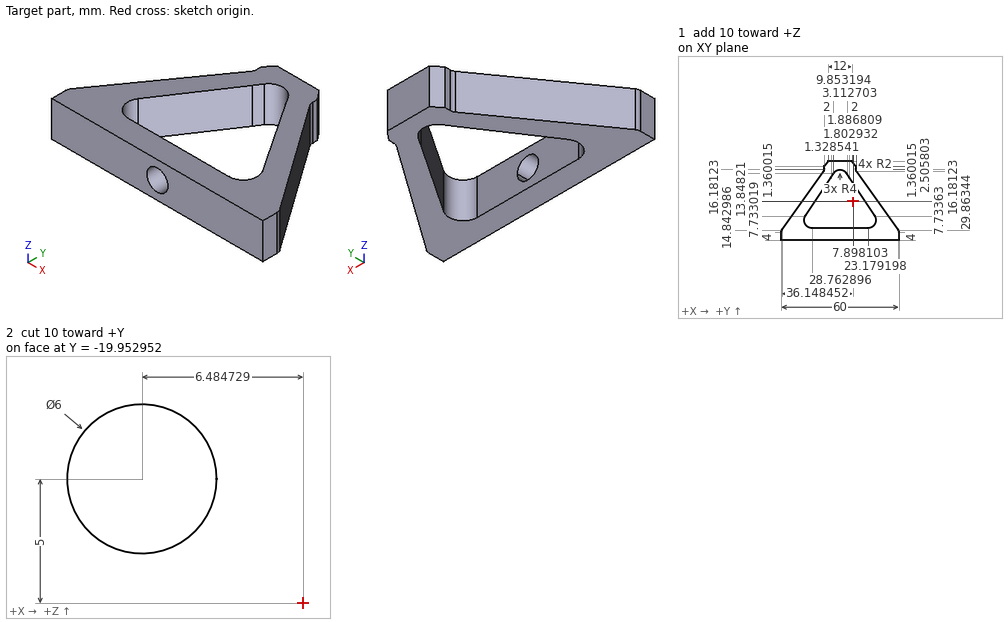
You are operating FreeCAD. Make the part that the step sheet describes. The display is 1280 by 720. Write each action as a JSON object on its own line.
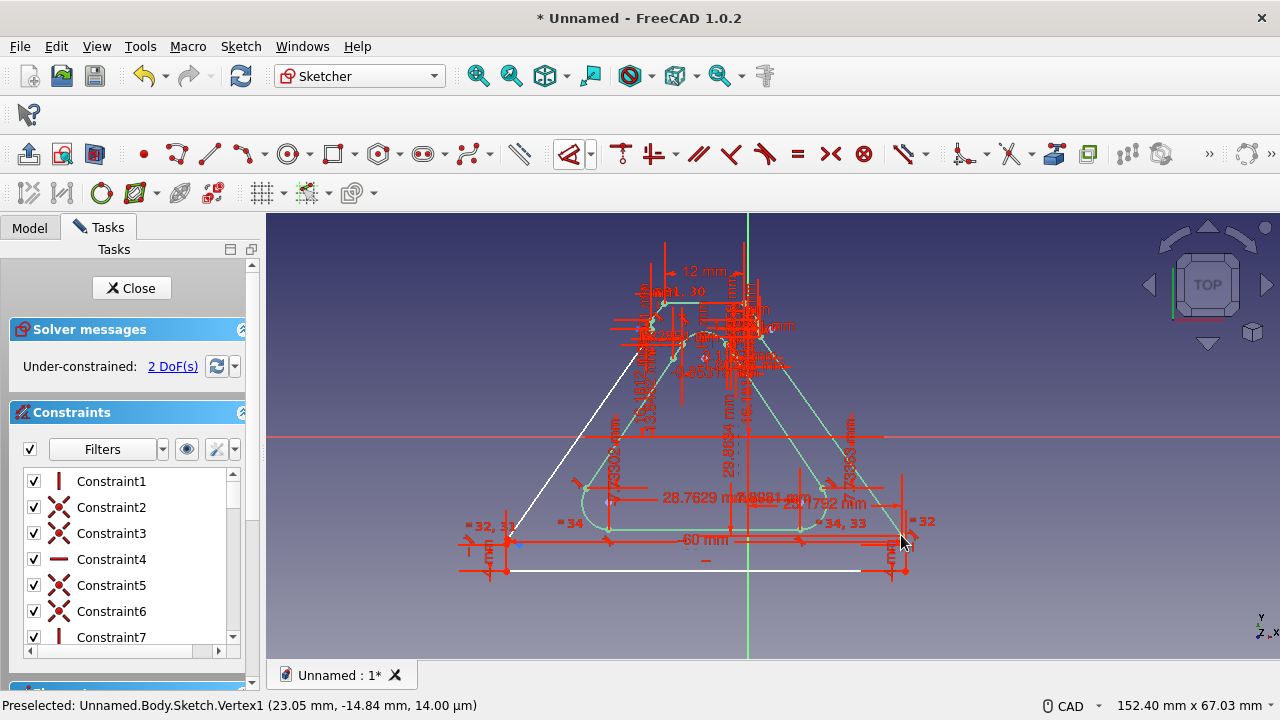
{"action": "scroll", "coordinate": [508, 540], "scroll_direction": "up", "scroll_amount": 5}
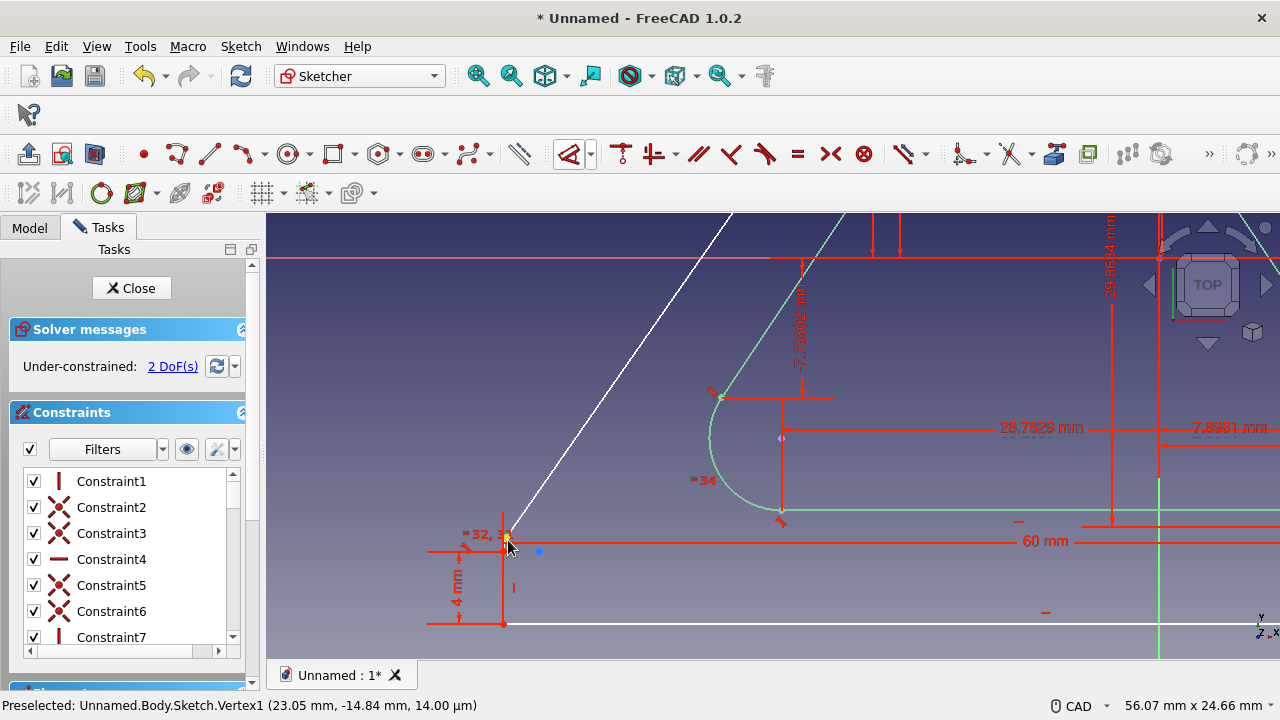
{"action": "left_click", "coordinate": [506, 538]}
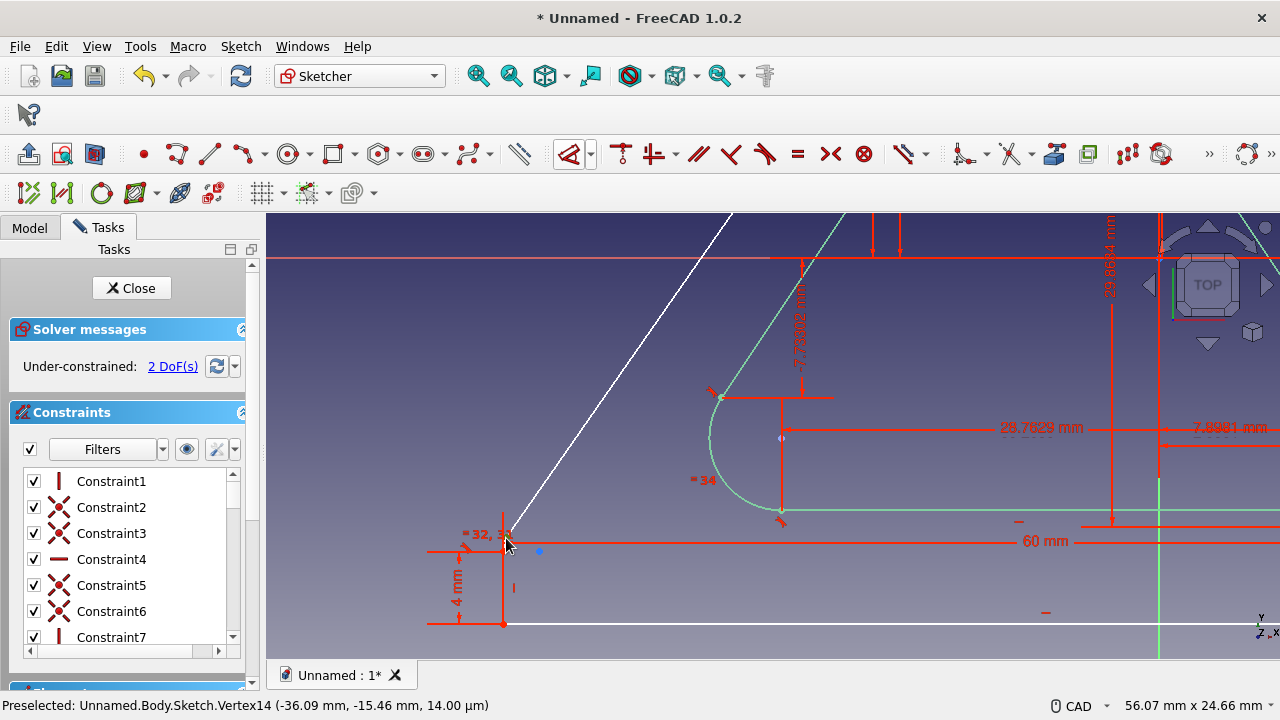
{"action": "left_click", "coordinate": [590, 154]}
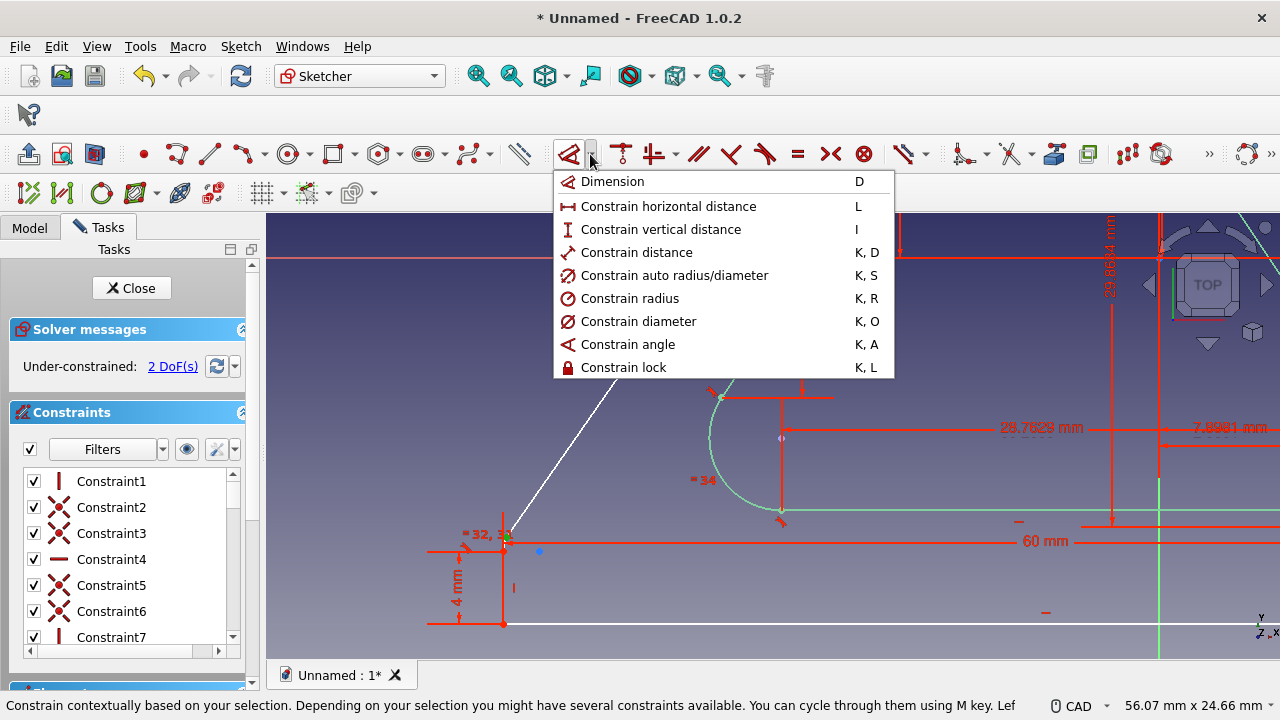
{"action": "left_click", "coordinate": [724, 206]}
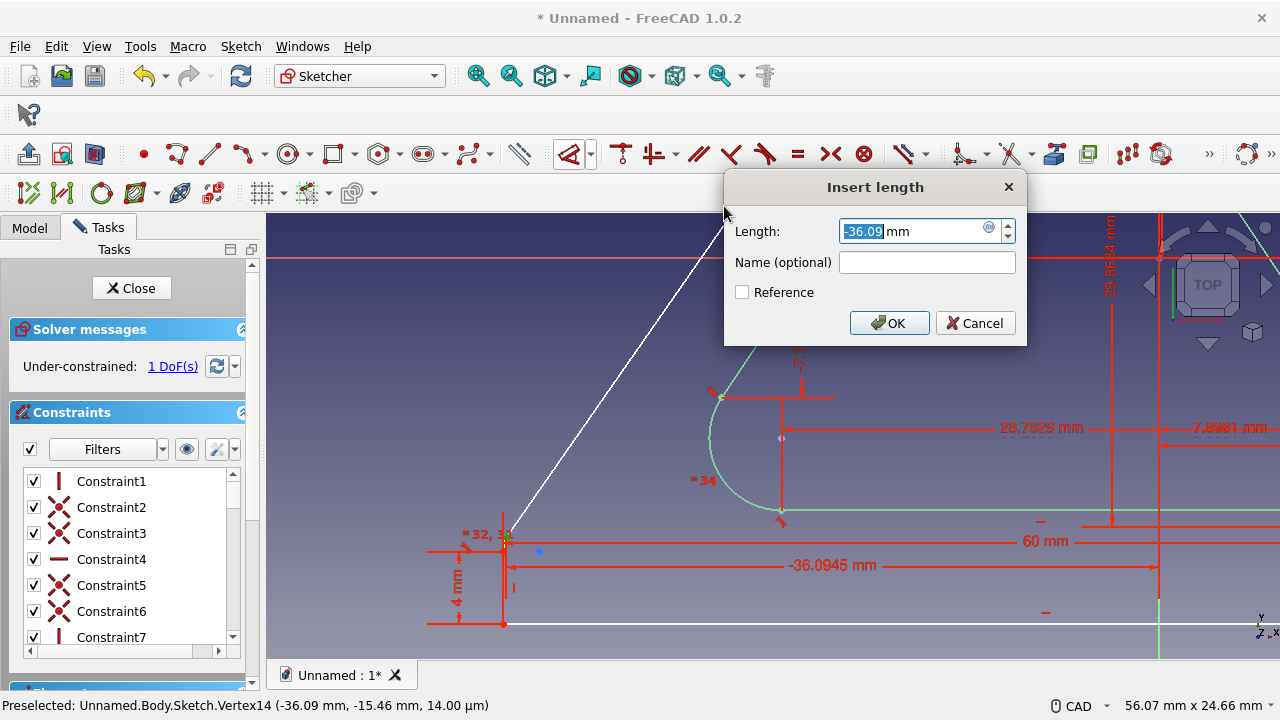
{"action": "type", "text": "-36.148452"}
{"action": "key", "text": "Return"}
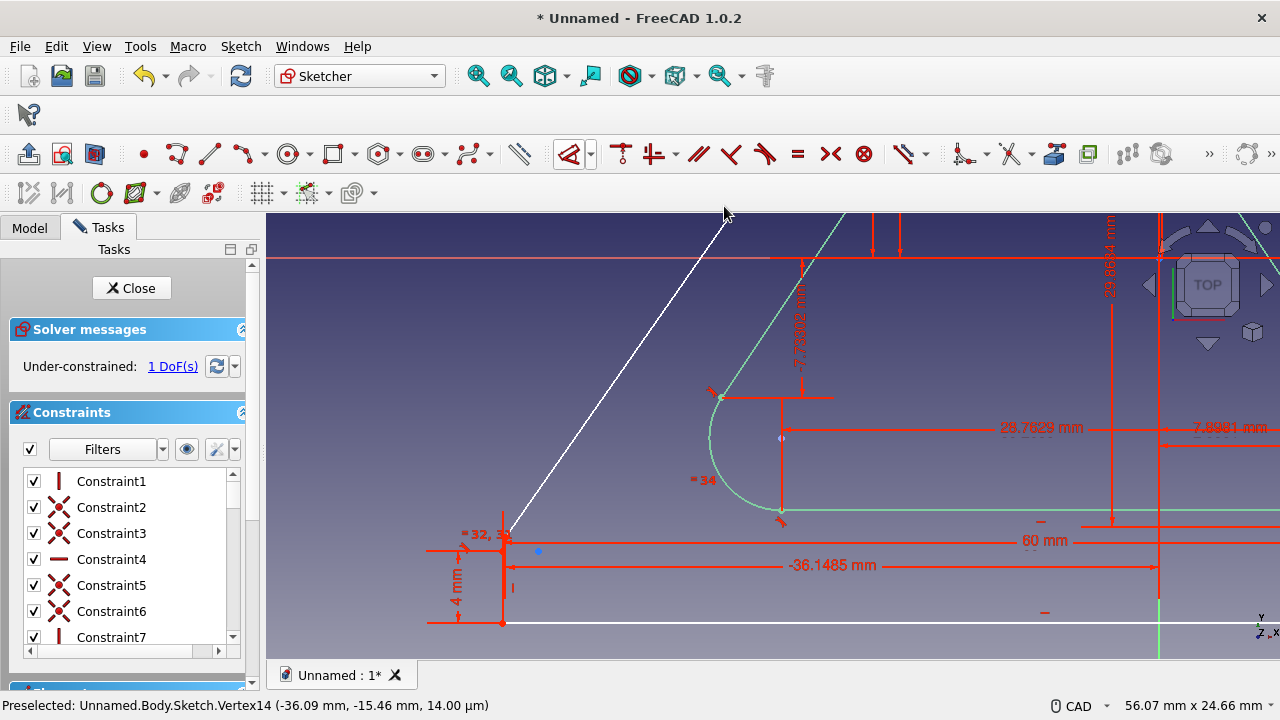
{"action": "left_click", "coordinate": [505, 538]}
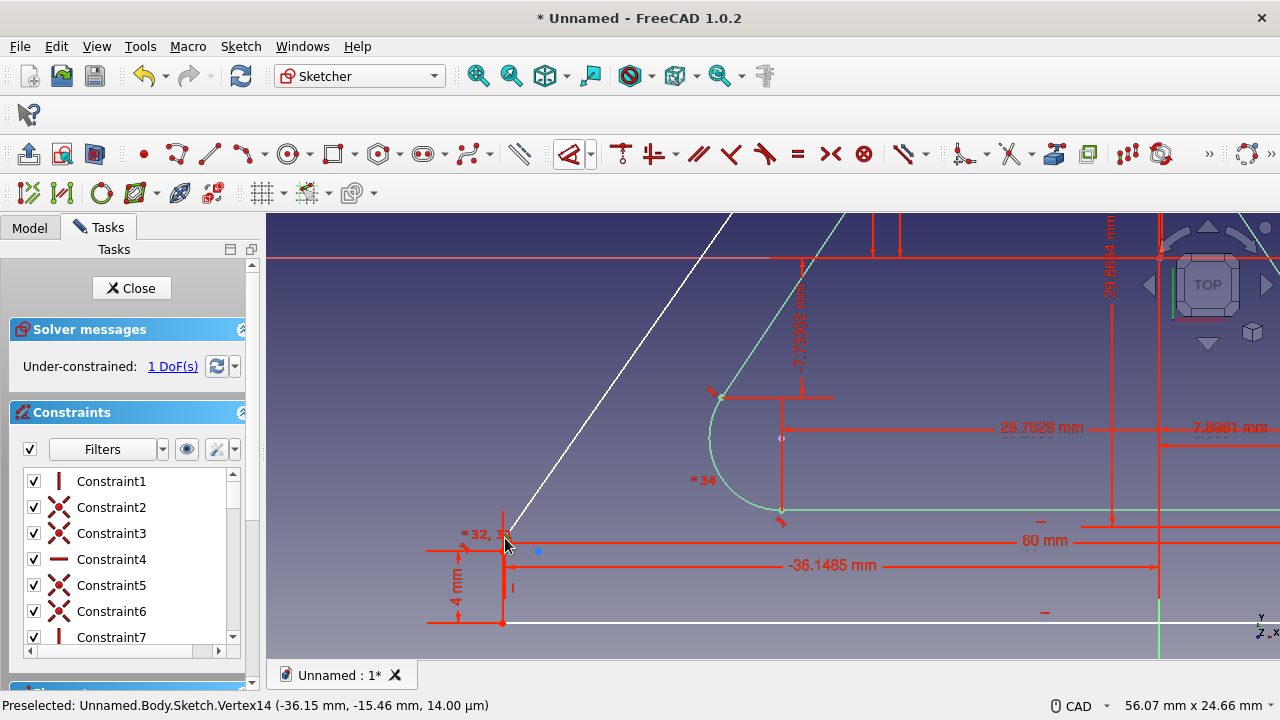
{"action": "left_click", "coordinate": [590, 154]}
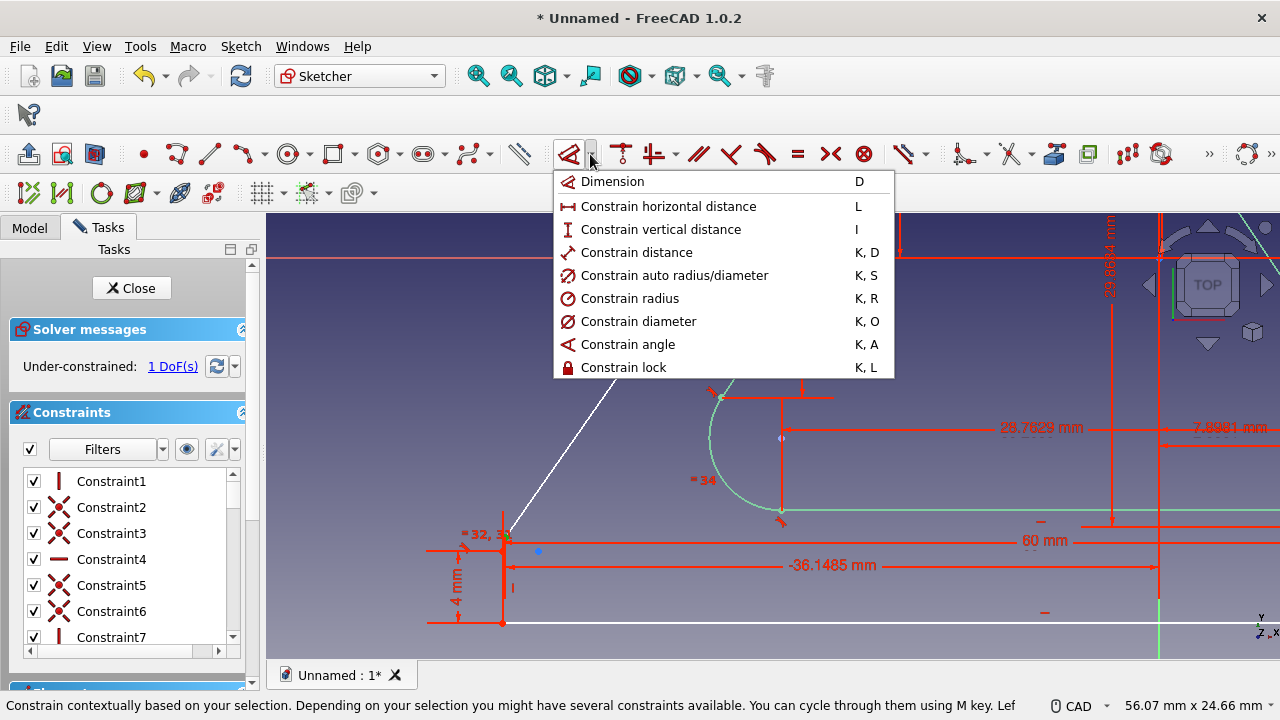
{"action": "left_click", "coordinate": [724, 230]}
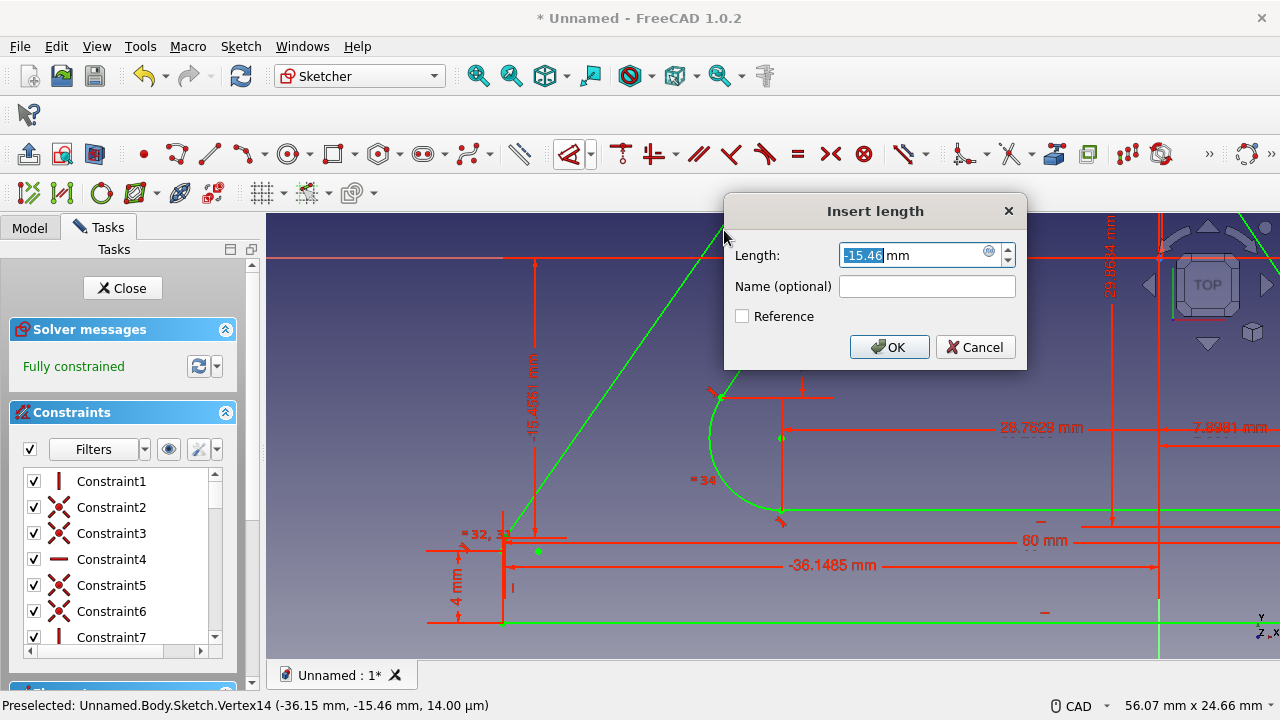
{"action": "type", "text": "-14.842986"}
{"action": "key", "text": "Return"}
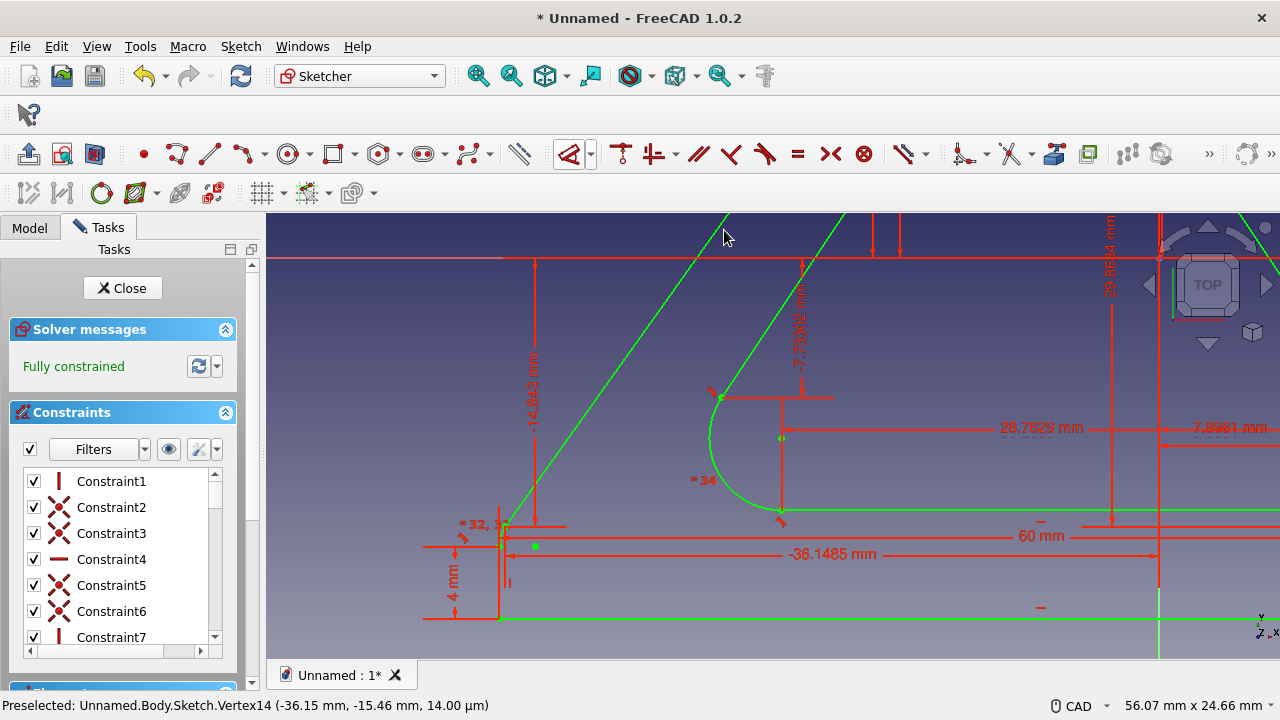
{"action": "left_click", "coordinate": [123, 288]}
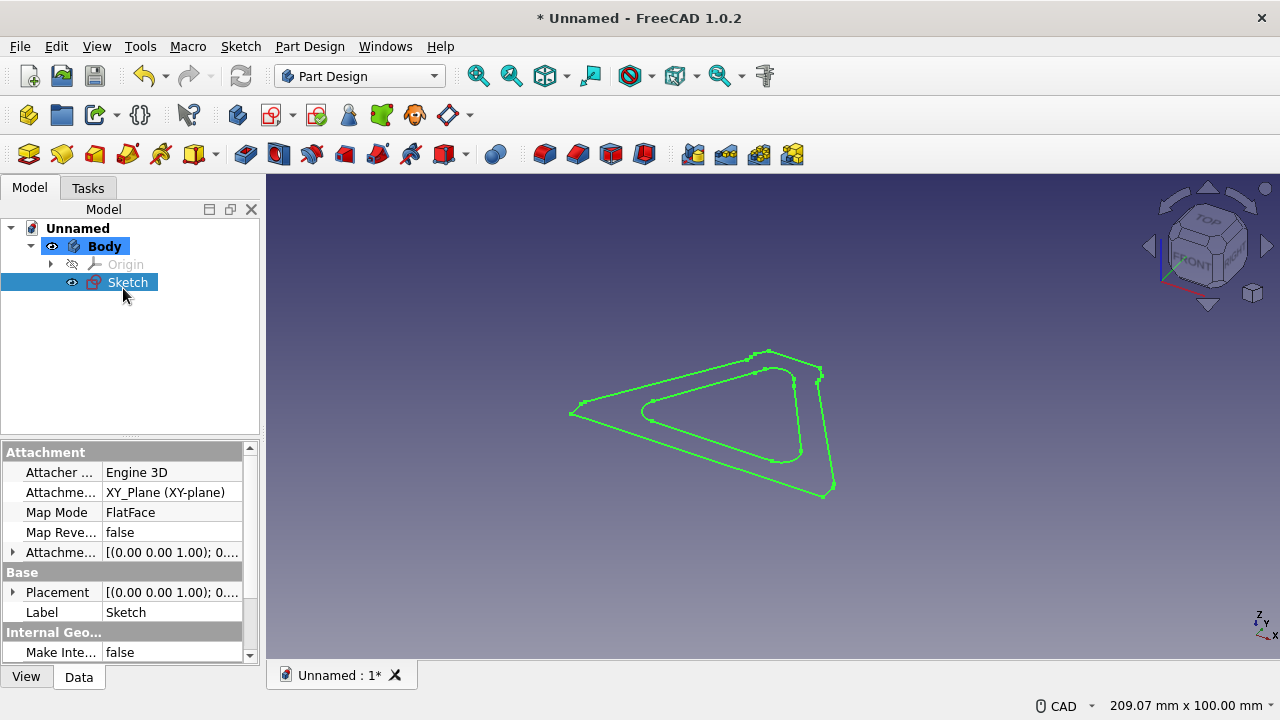
{"action": "left_click", "coordinate": [29, 154]}